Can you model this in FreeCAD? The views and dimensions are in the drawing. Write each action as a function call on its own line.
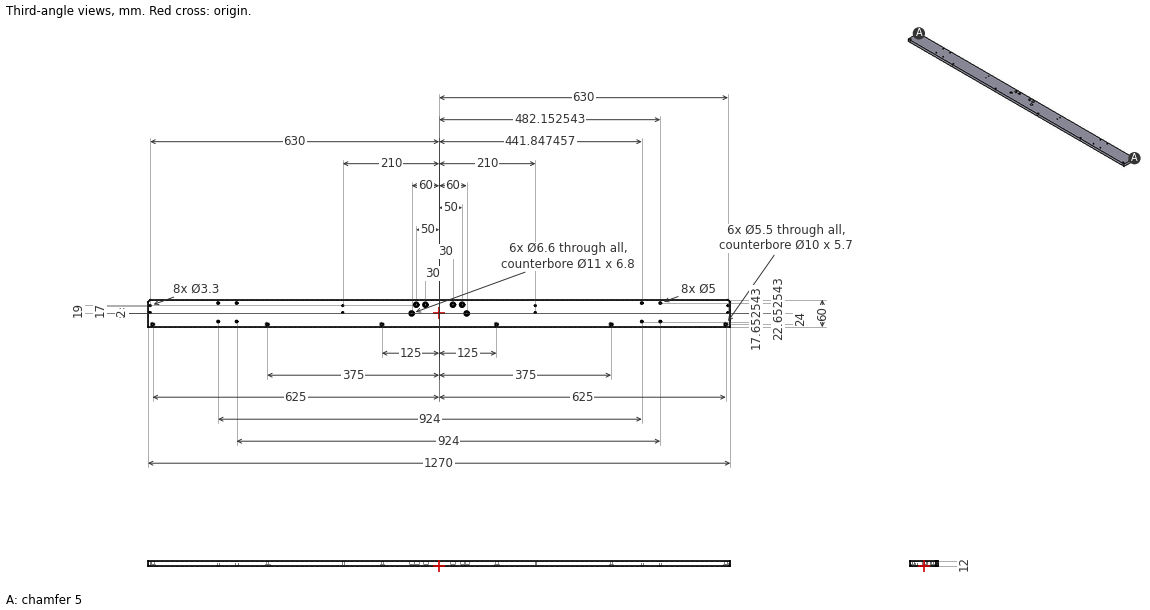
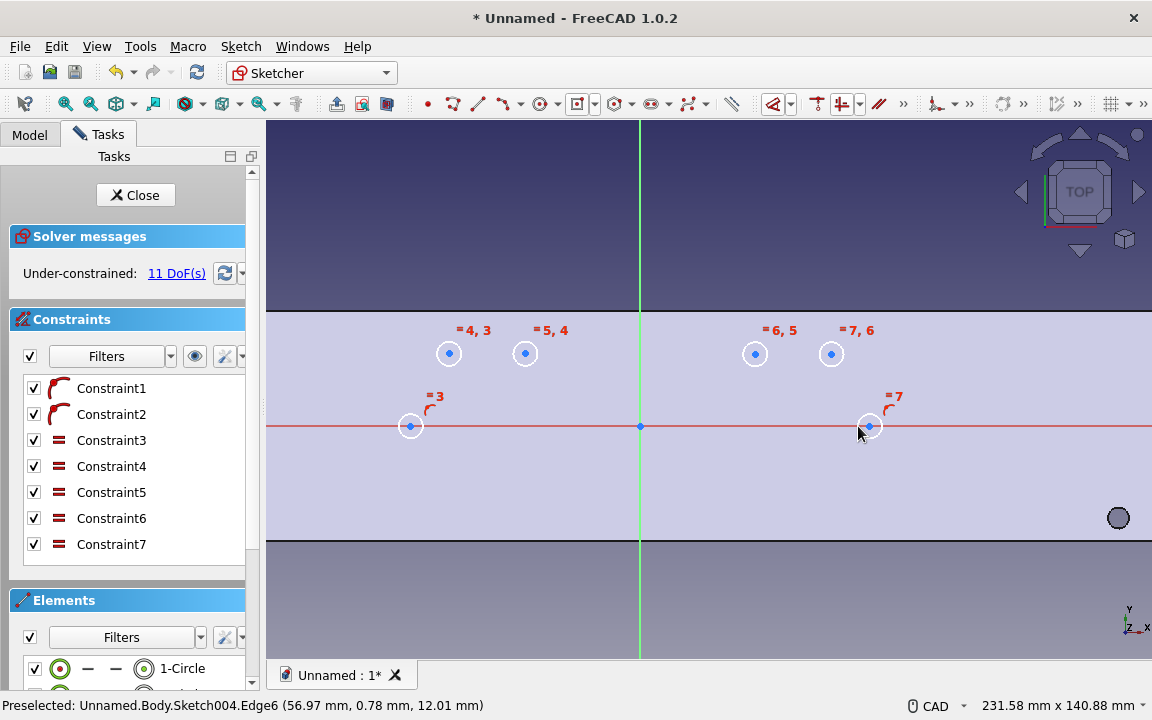
click(449, 354)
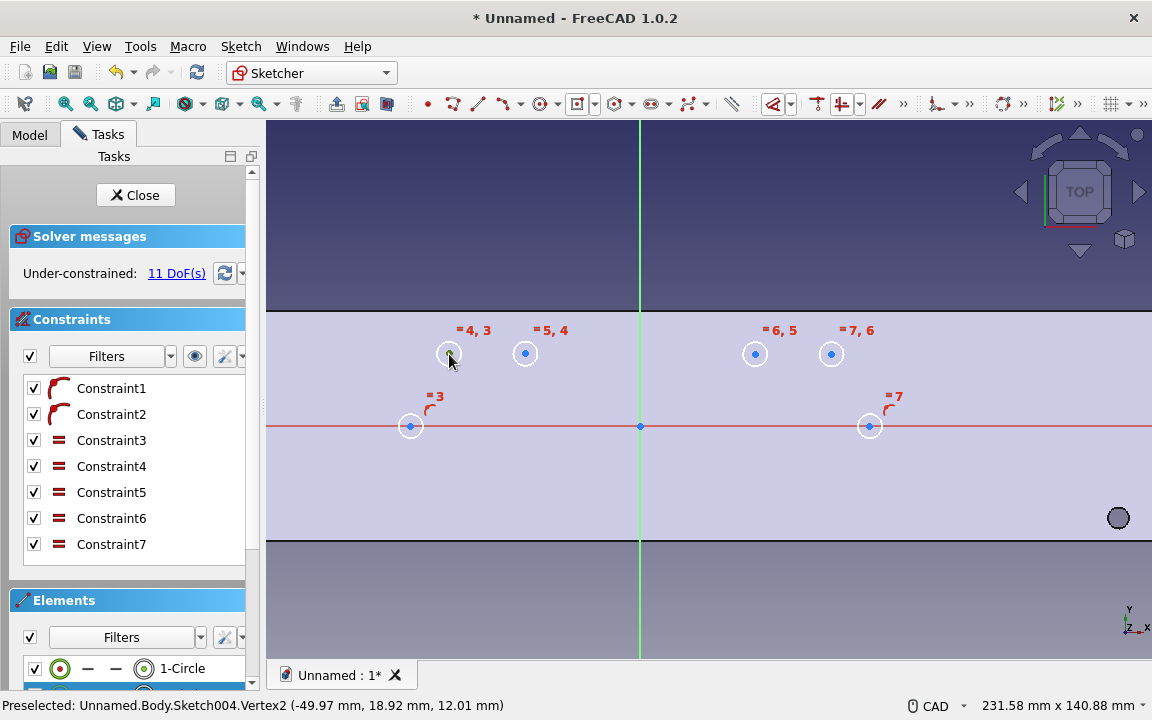
click(525, 354)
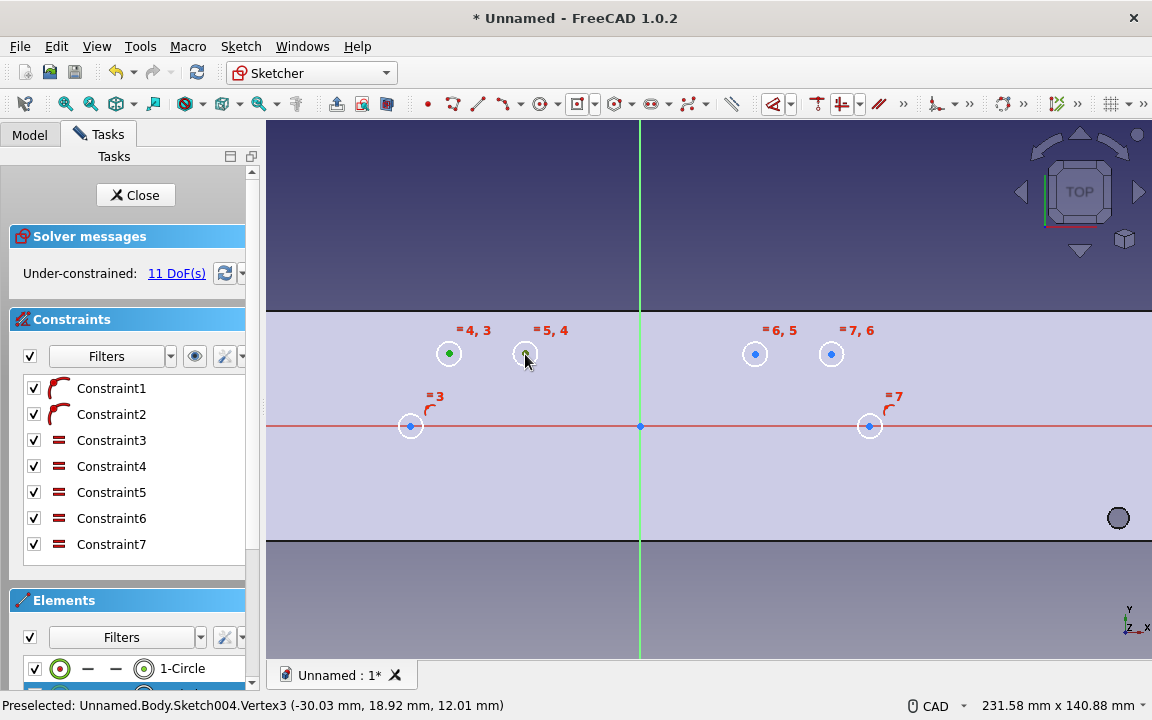
click(860, 104)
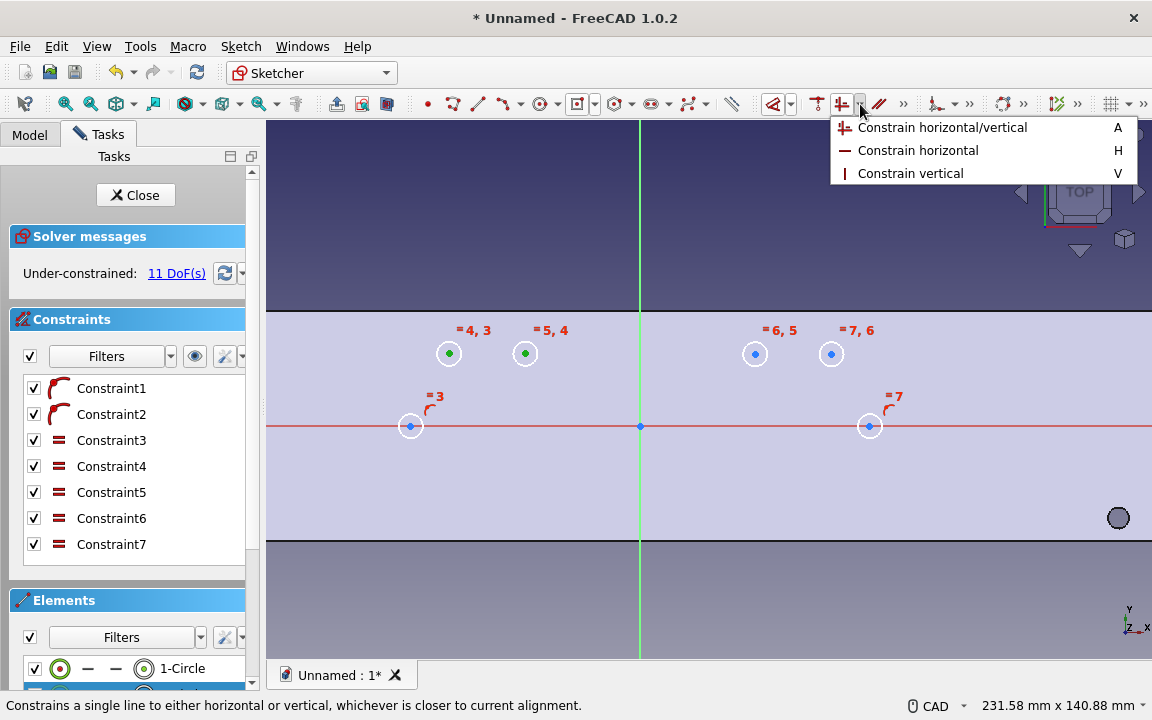
click(984, 150)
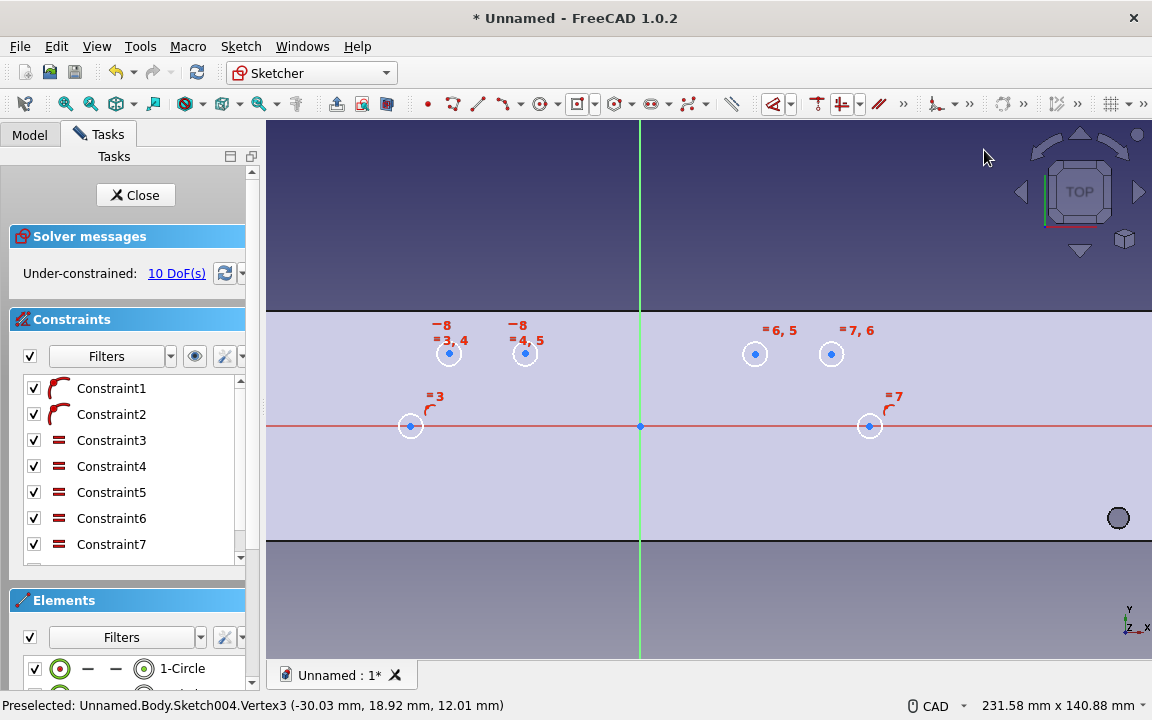
click(525, 354)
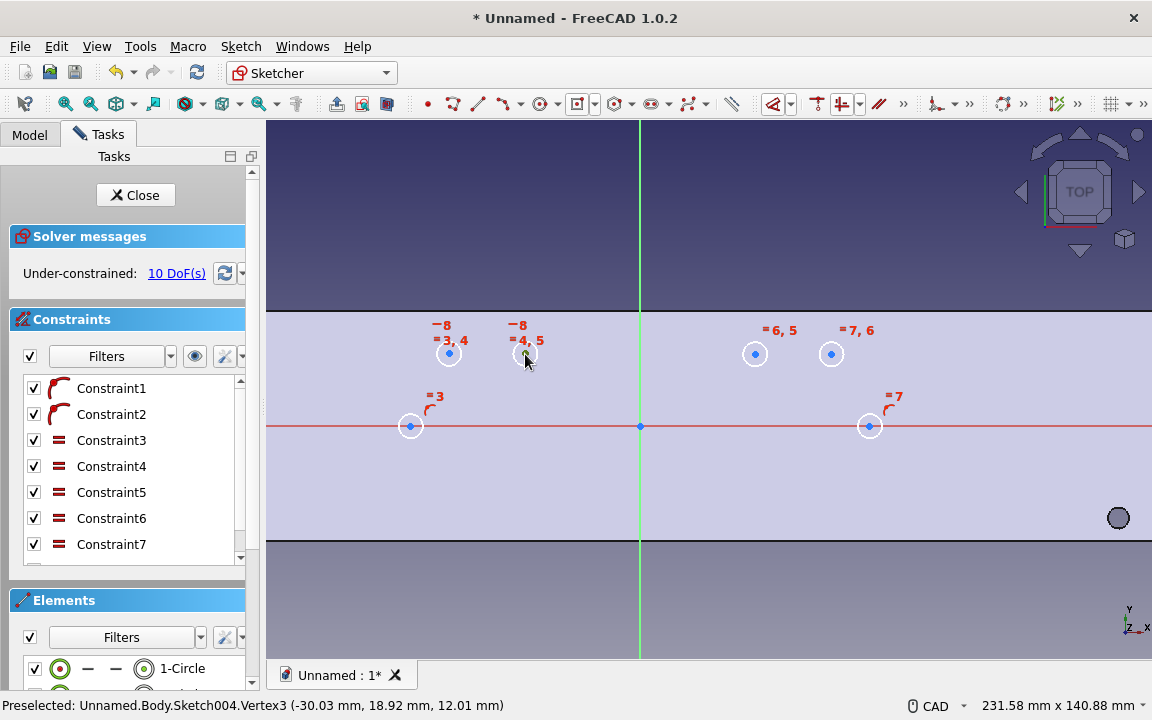
click(755, 354)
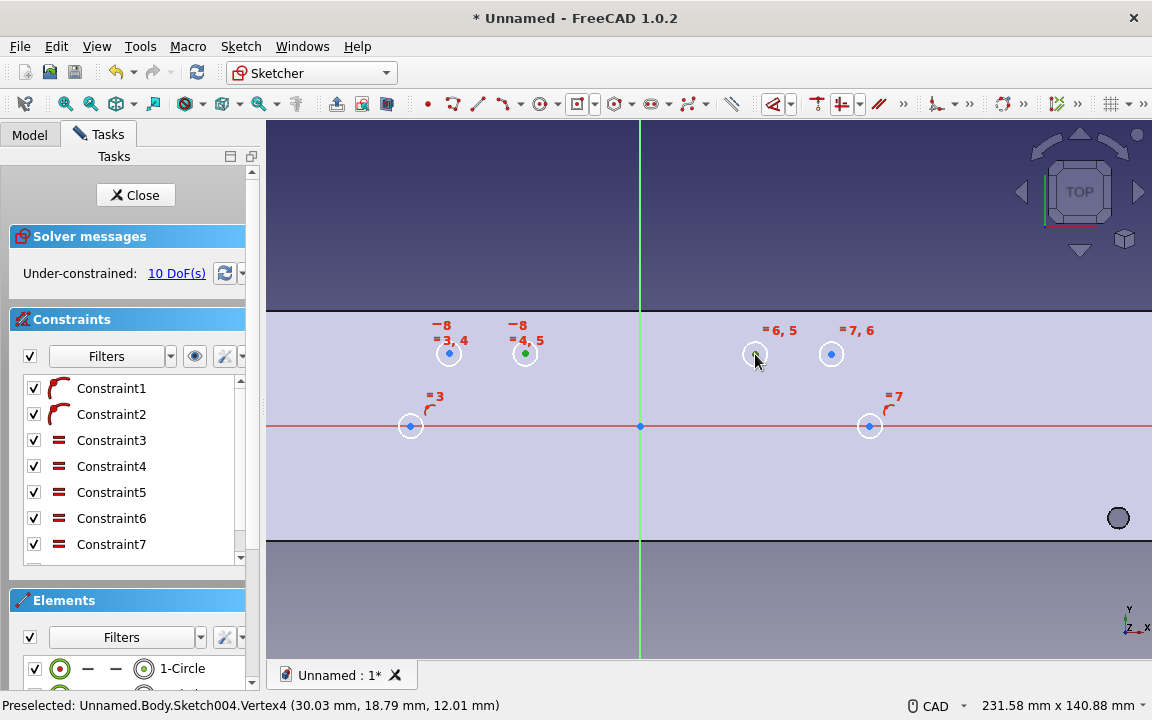
key(h)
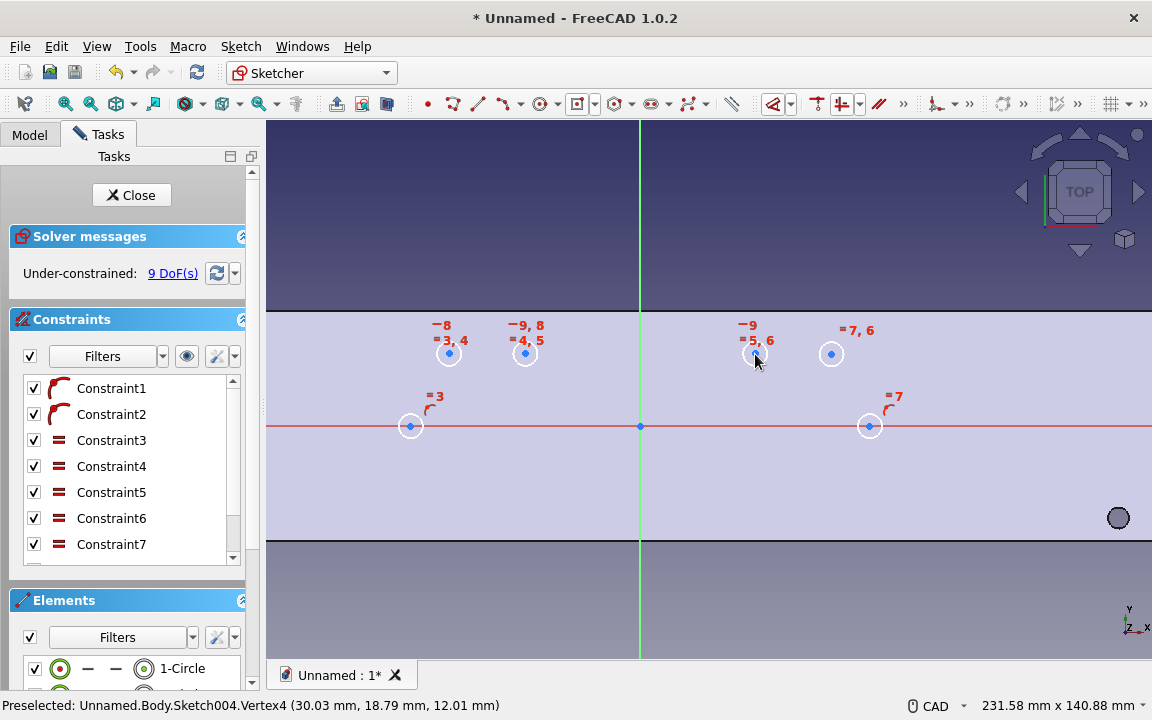
click(755, 354)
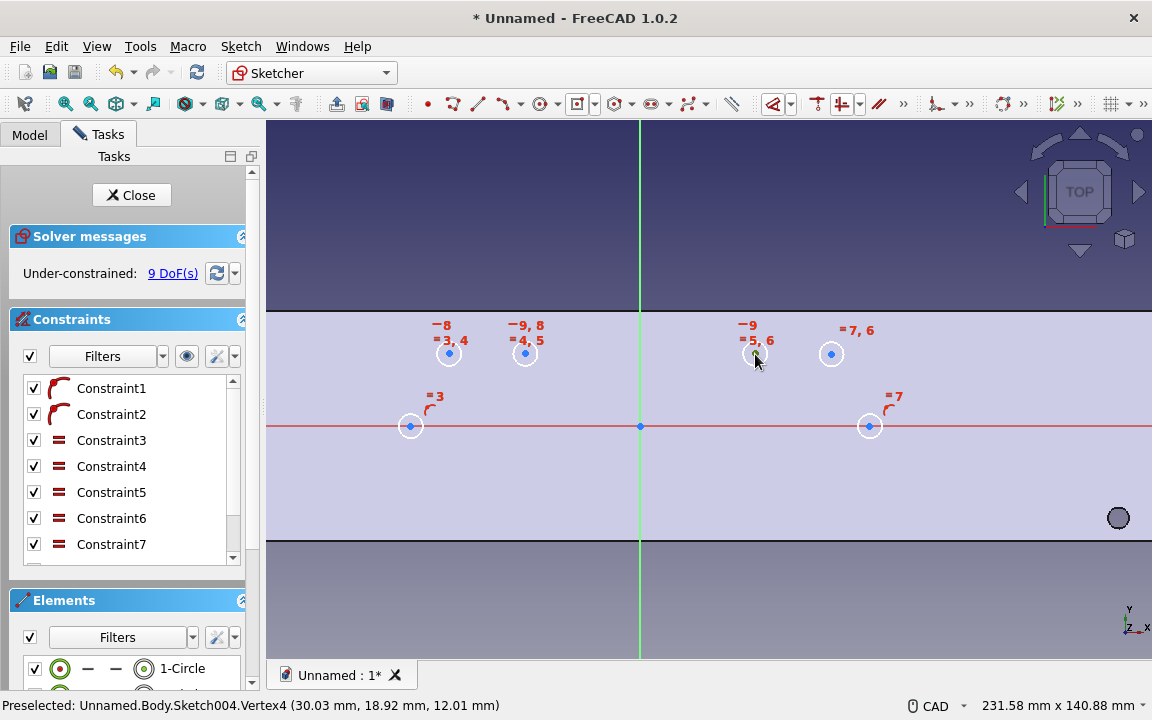
click(832, 354)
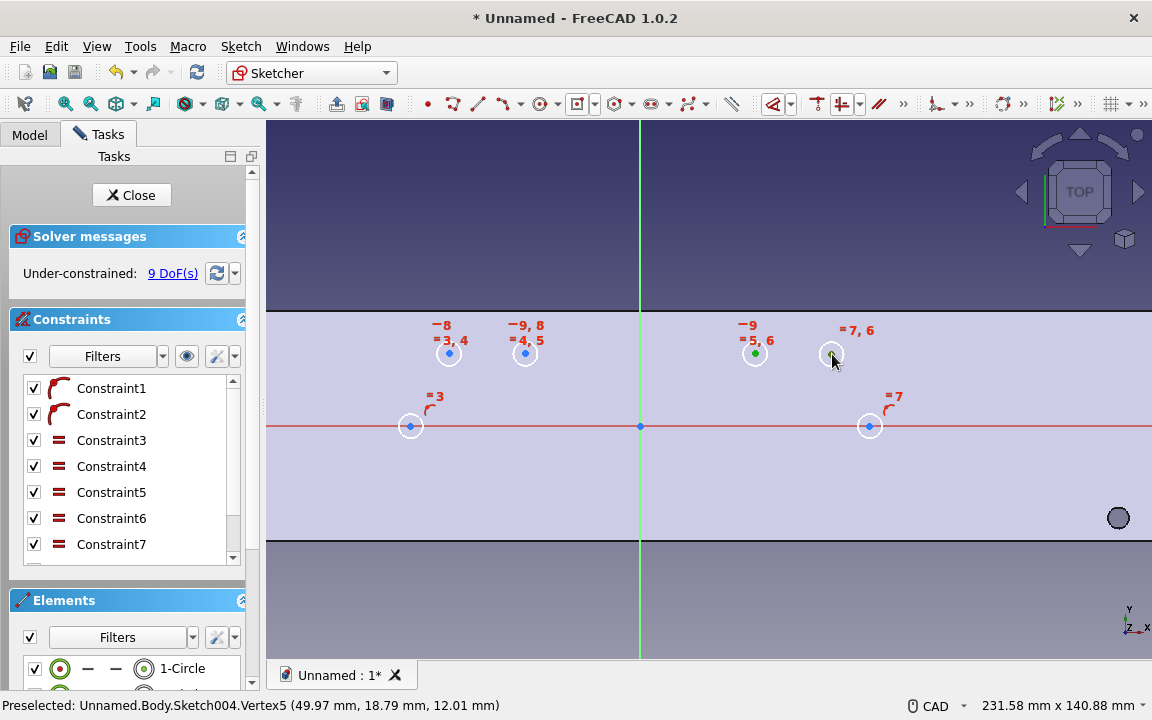
click(860, 104)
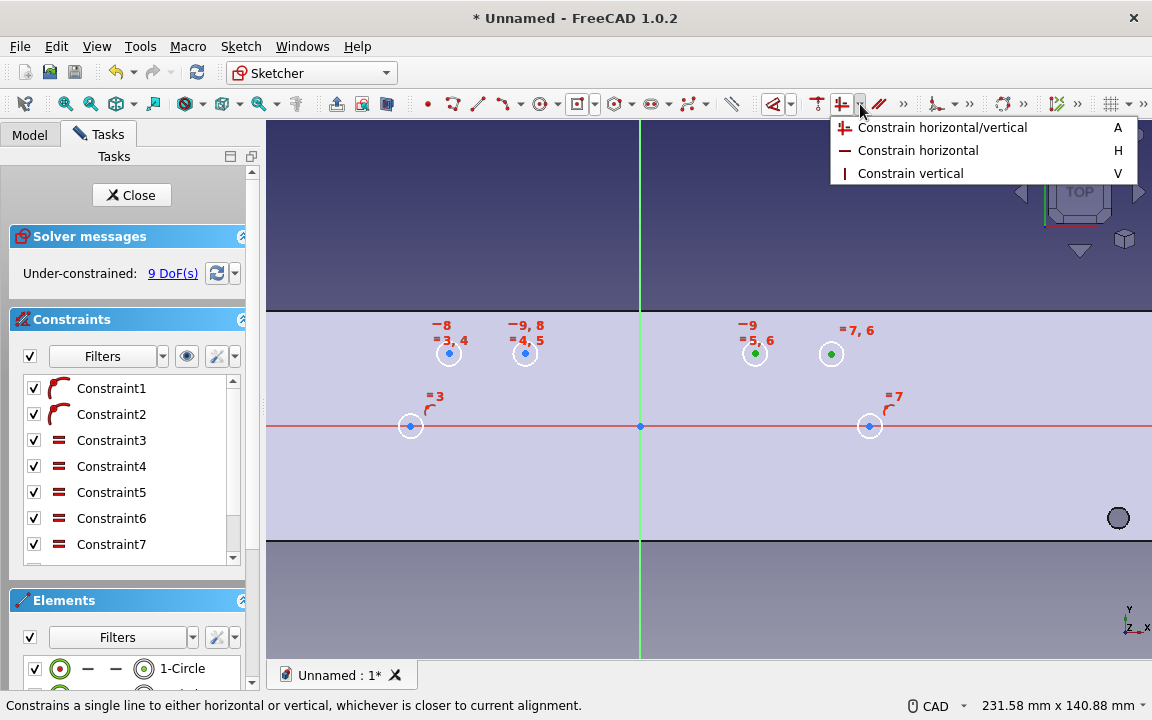
click(984, 150)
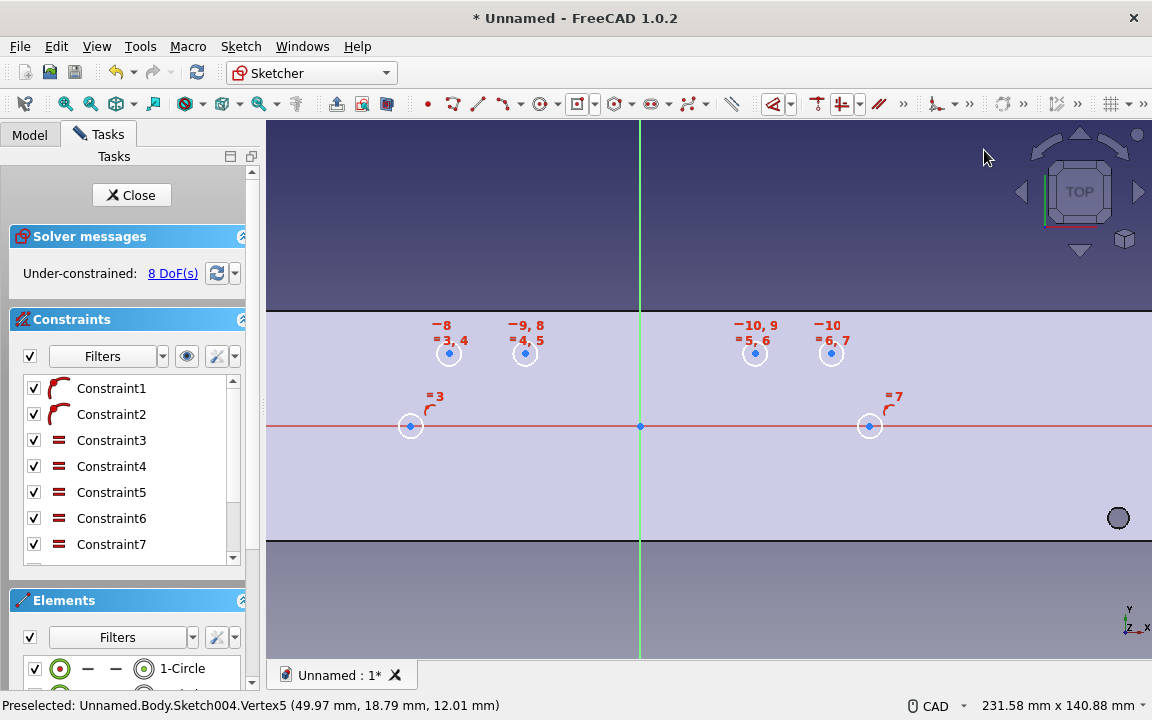
scroll(411, 414, up, 3)